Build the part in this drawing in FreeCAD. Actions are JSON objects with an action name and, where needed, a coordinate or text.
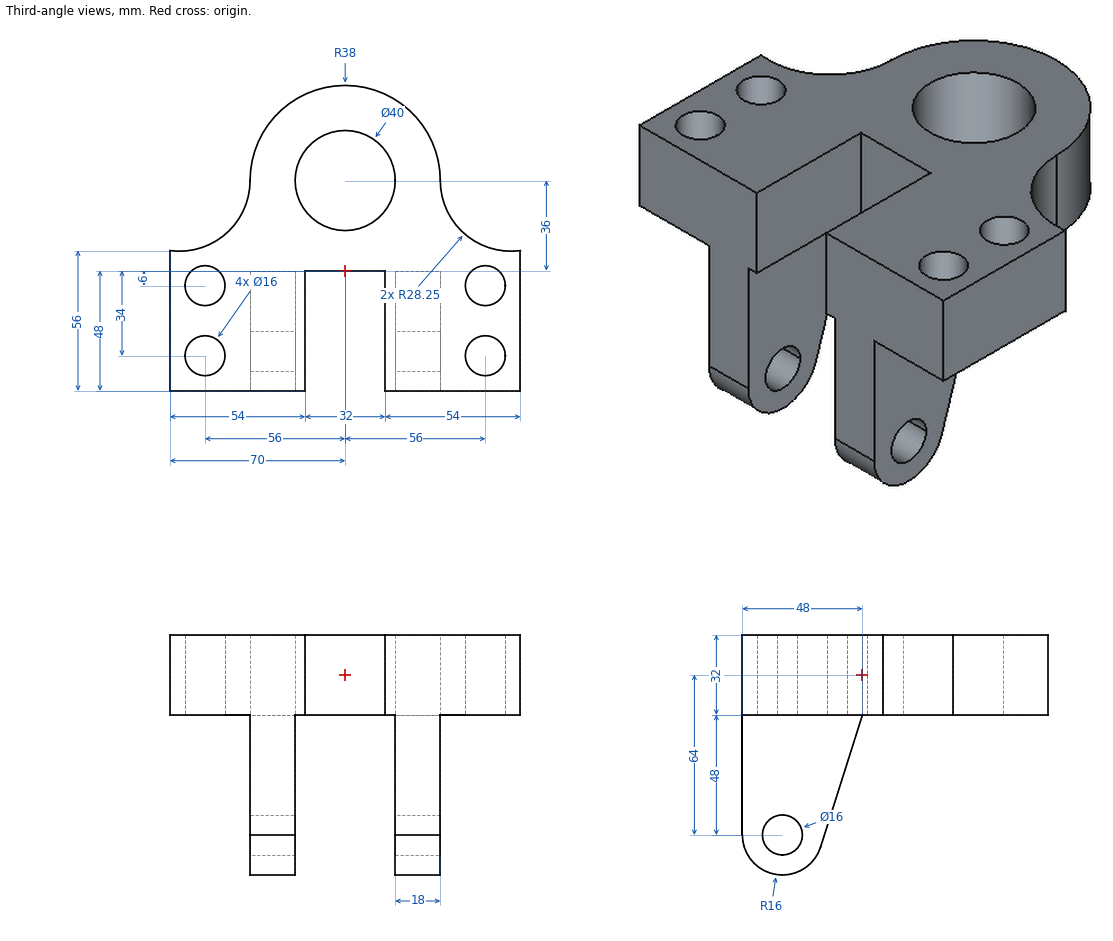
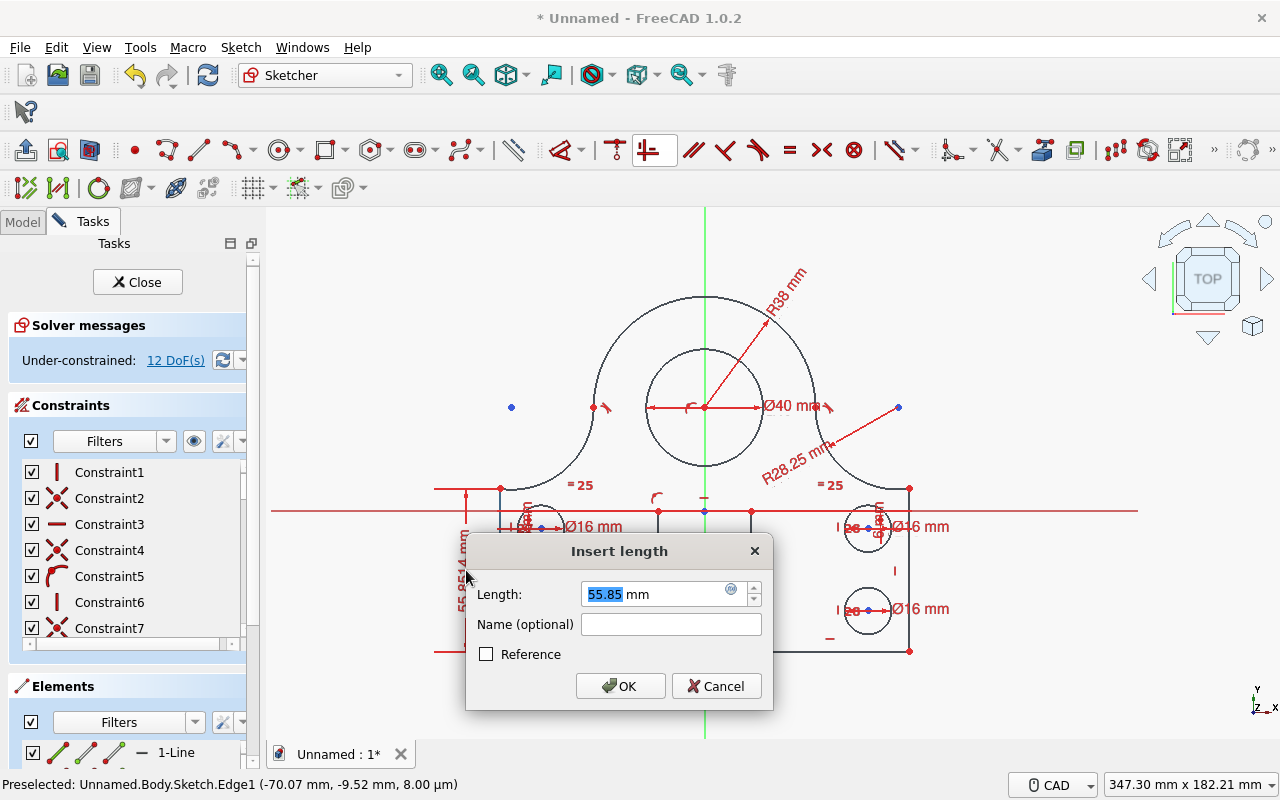
{"action": "type", "text": "56"}
{"action": "key", "text": "Return"}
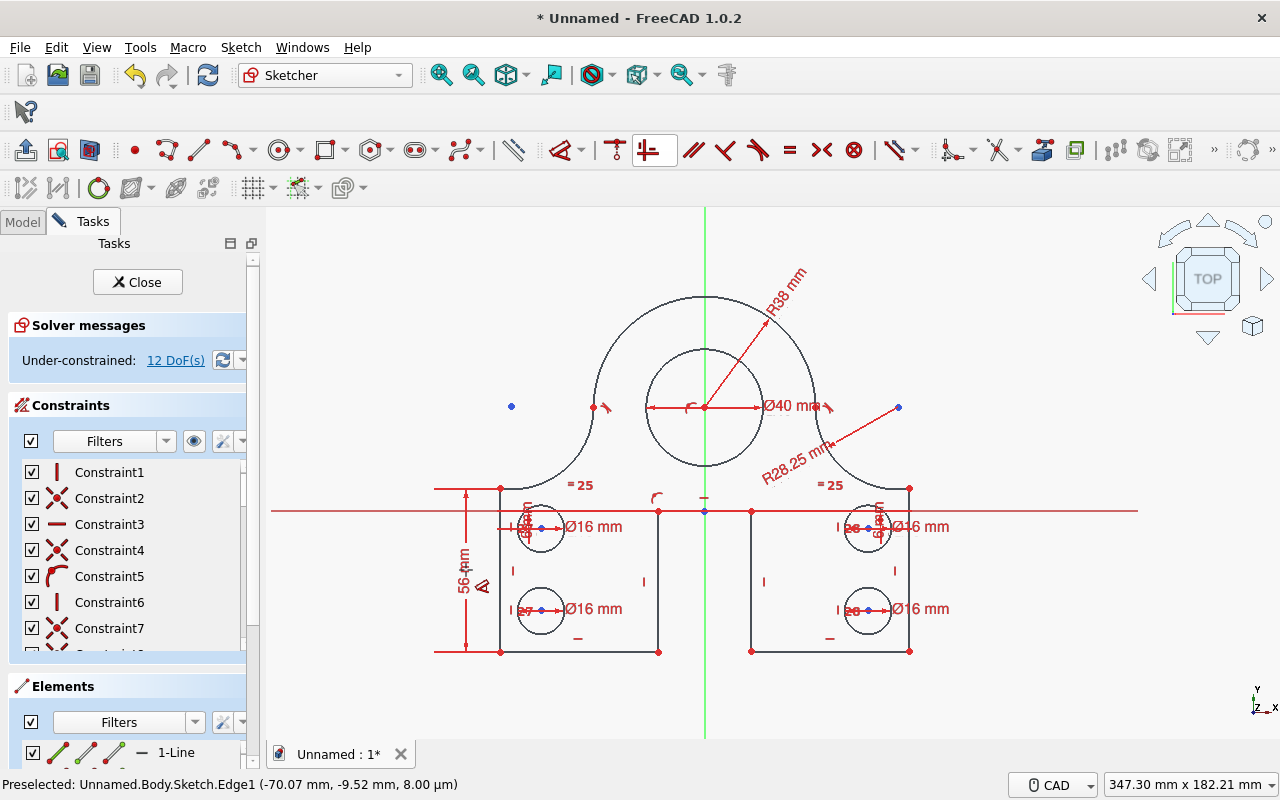
{"action": "left_click", "coordinate": [547, 652]}
{"action": "left_click", "coordinate": [579, 686]}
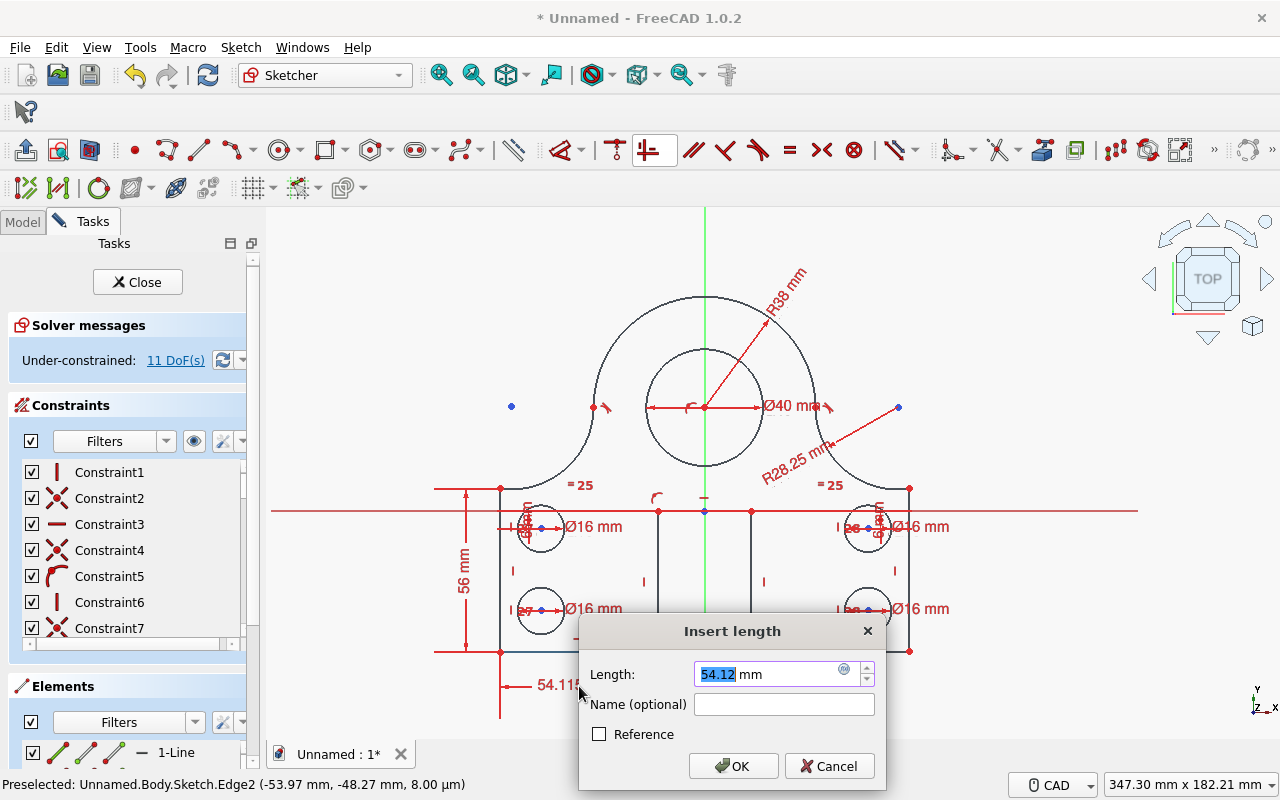
{"action": "type", "text": "54"}
{"action": "key", "text": "Return"}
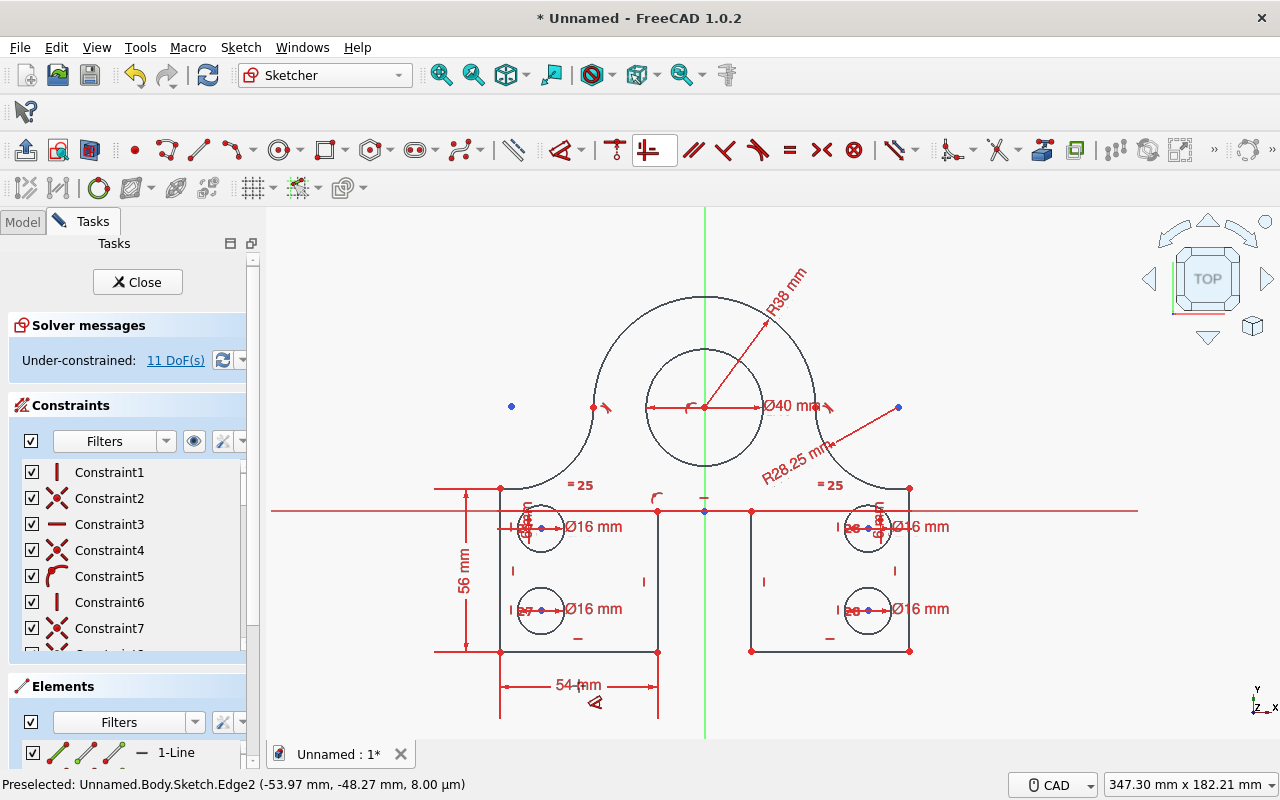
{"action": "left_click", "coordinate": [658, 610]}
{"action": "left_click", "coordinate": [624, 582]}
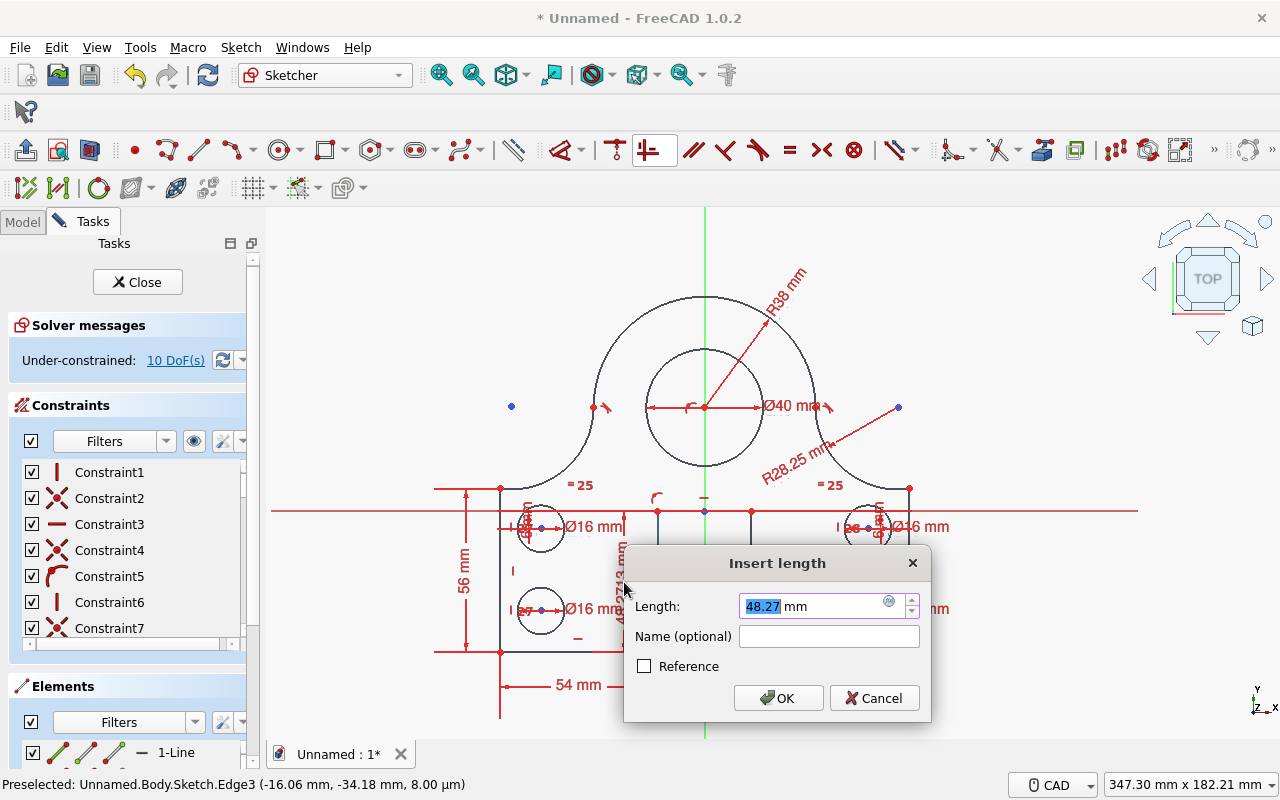
{"action": "type", "text": "48"}
{"action": "key", "text": "Return"}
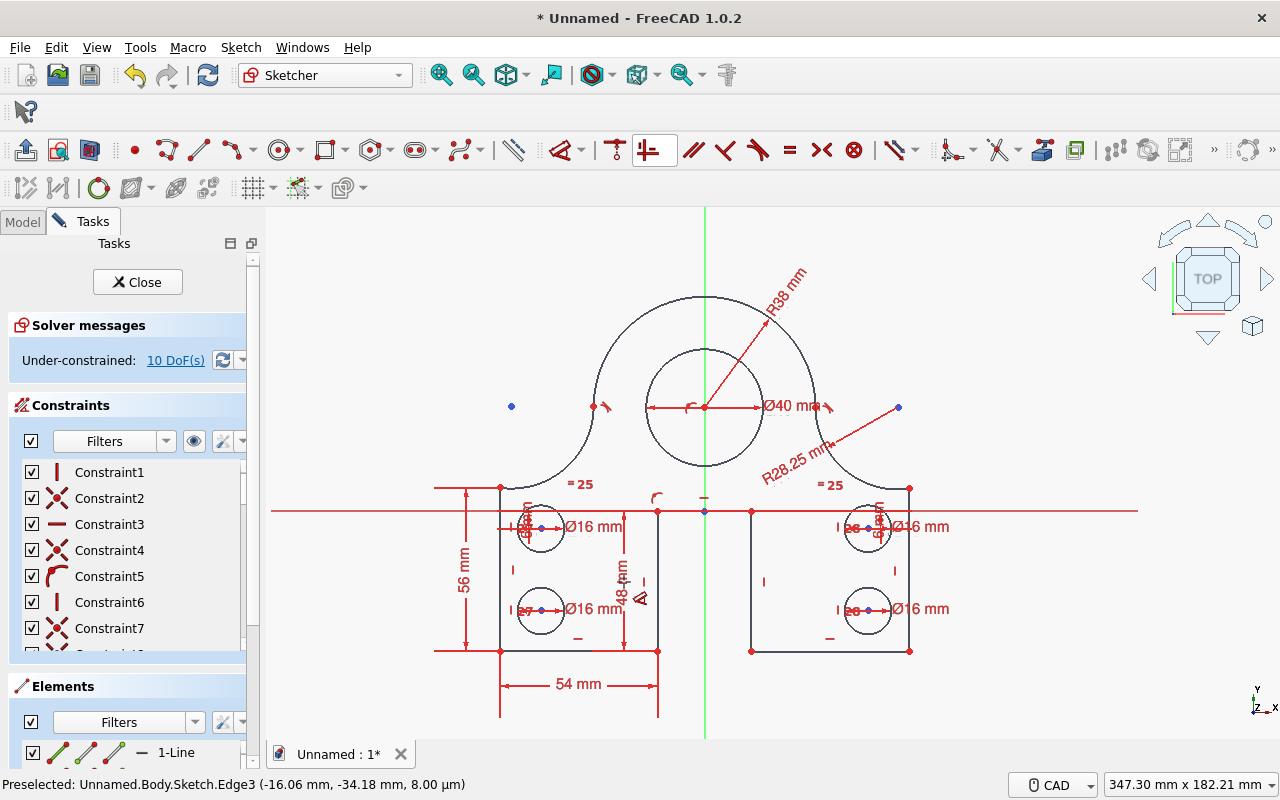
{"action": "left_click", "coordinate": [686, 511]}
{"action": "left_click", "coordinate": [683, 545]}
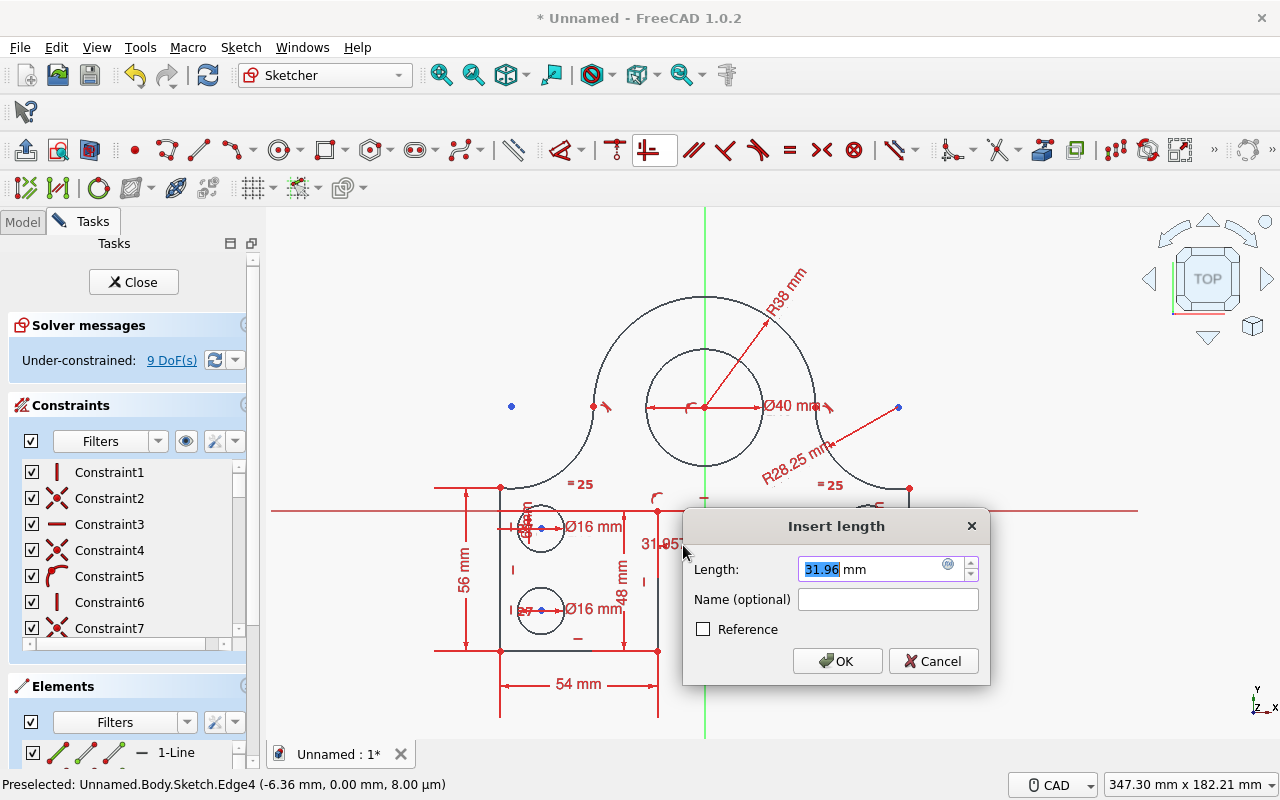
{"action": "type", "text": "32"}
{"action": "key", "text": "Return"}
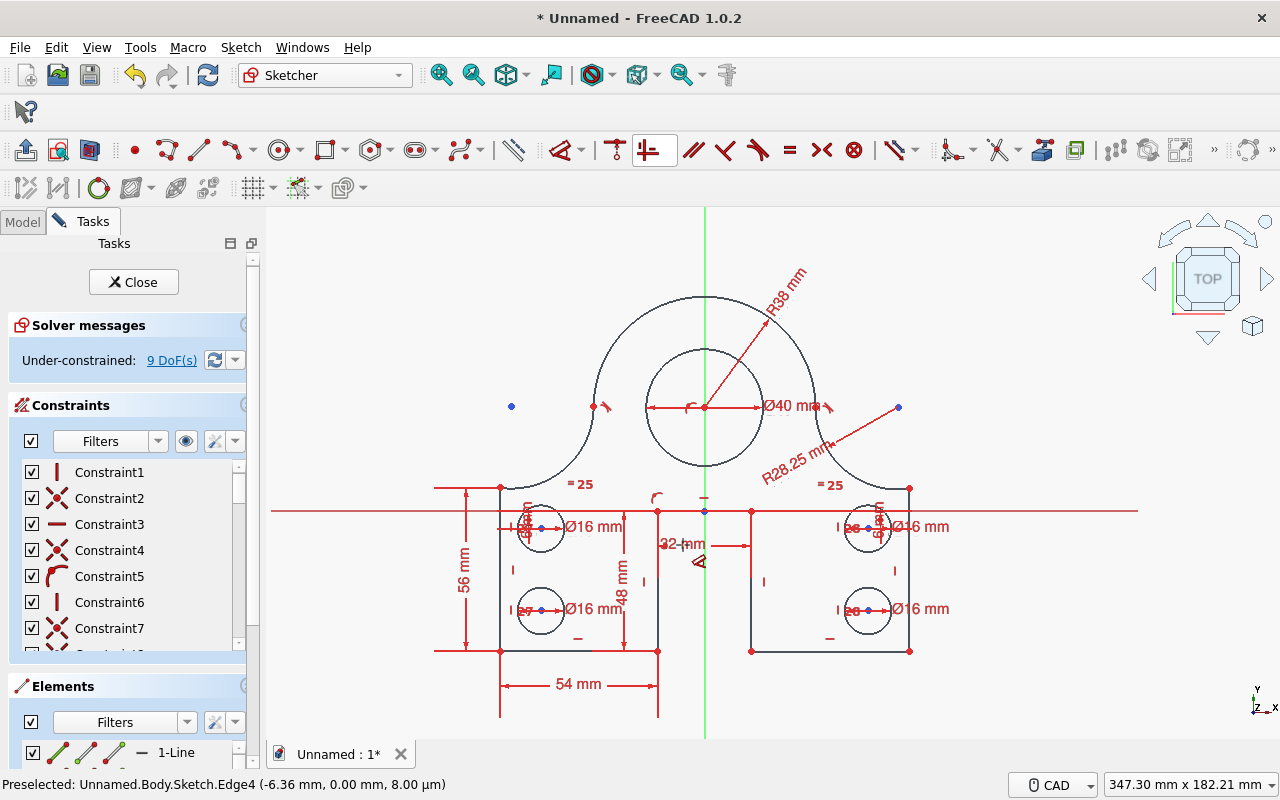
{"action": "left_click", "coordinate": [751, 553]}
{"action": "left_click", "coordinate": [785, 582]}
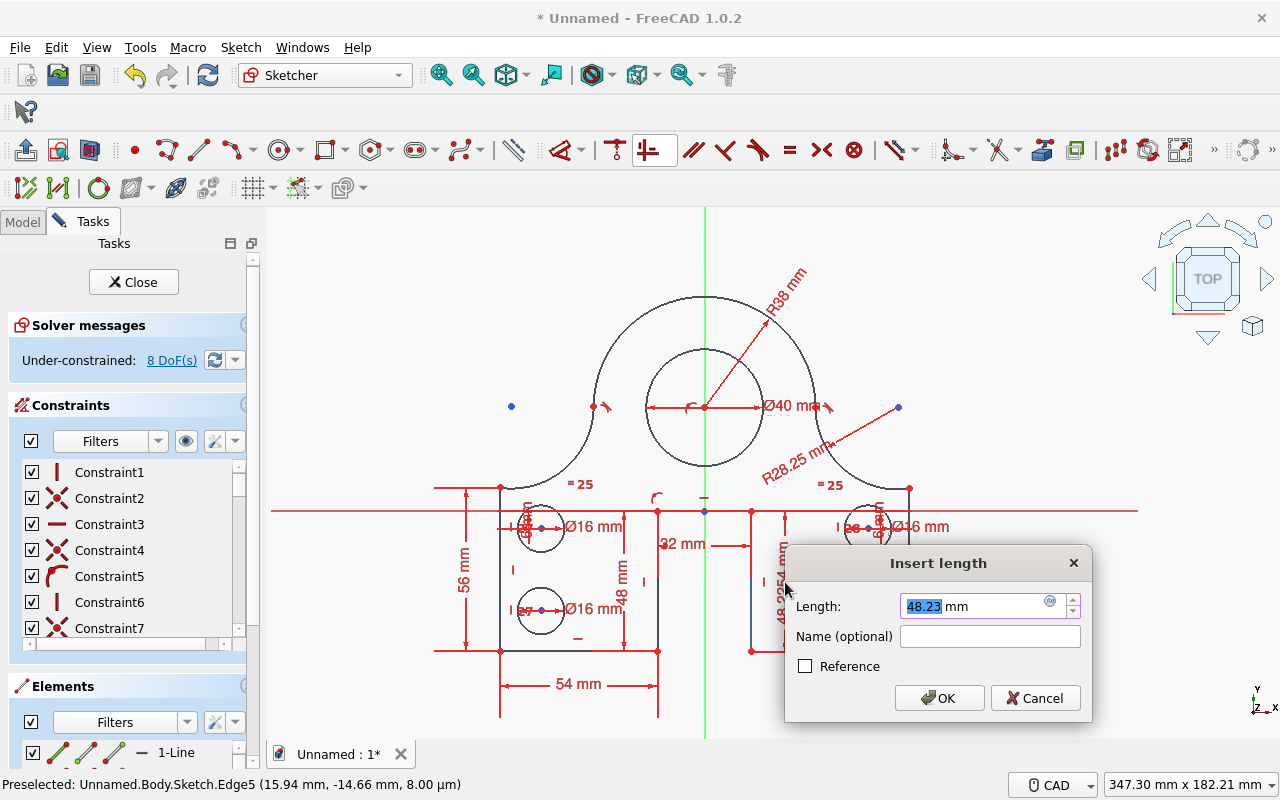
{"action": "type", "text": "48"}
{"action": "key", "text": "Return"}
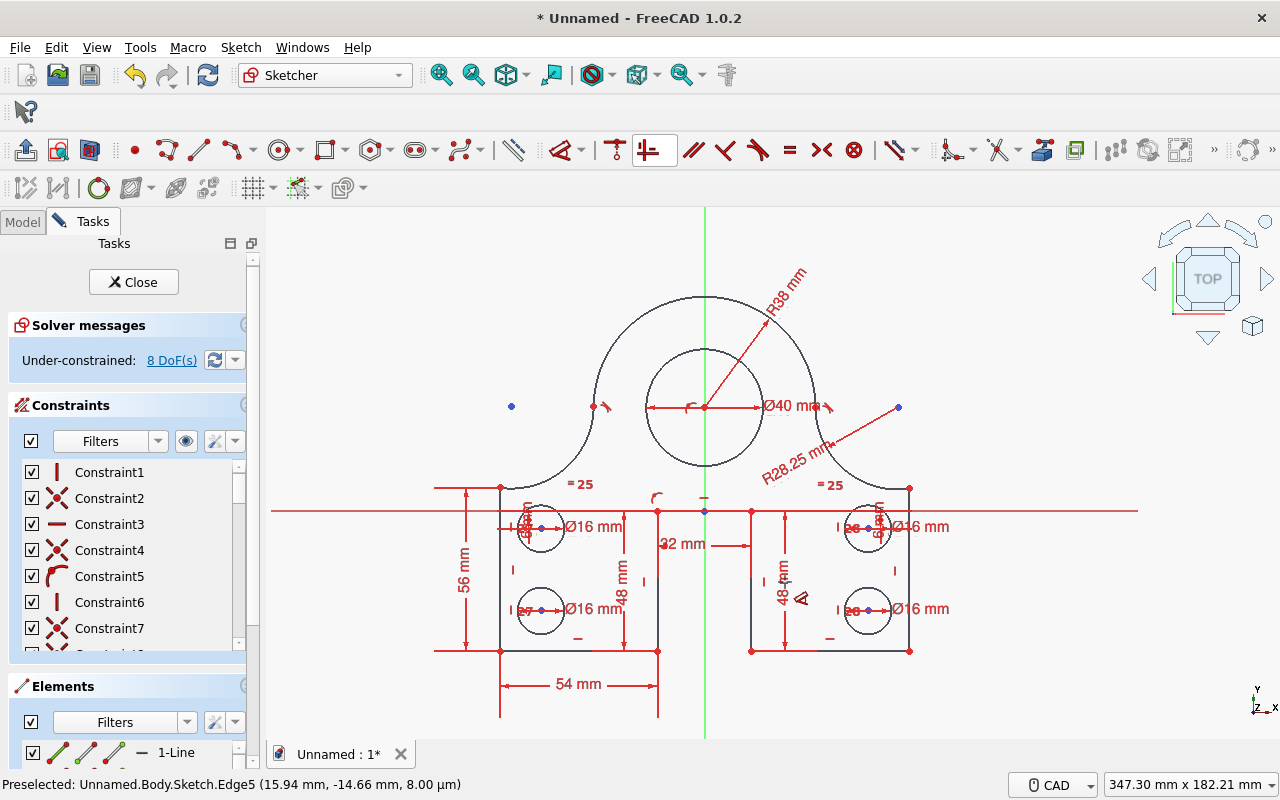
{"action": "left_click", "coordinate": [798, 651]}
{"action": "left_click", "coordinate": [830, 685]}